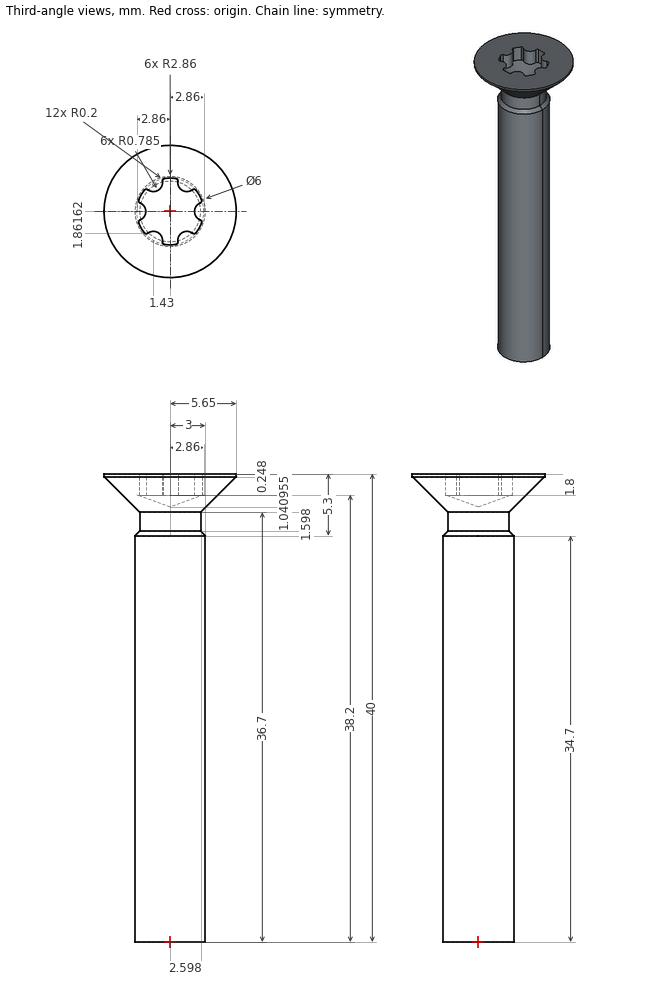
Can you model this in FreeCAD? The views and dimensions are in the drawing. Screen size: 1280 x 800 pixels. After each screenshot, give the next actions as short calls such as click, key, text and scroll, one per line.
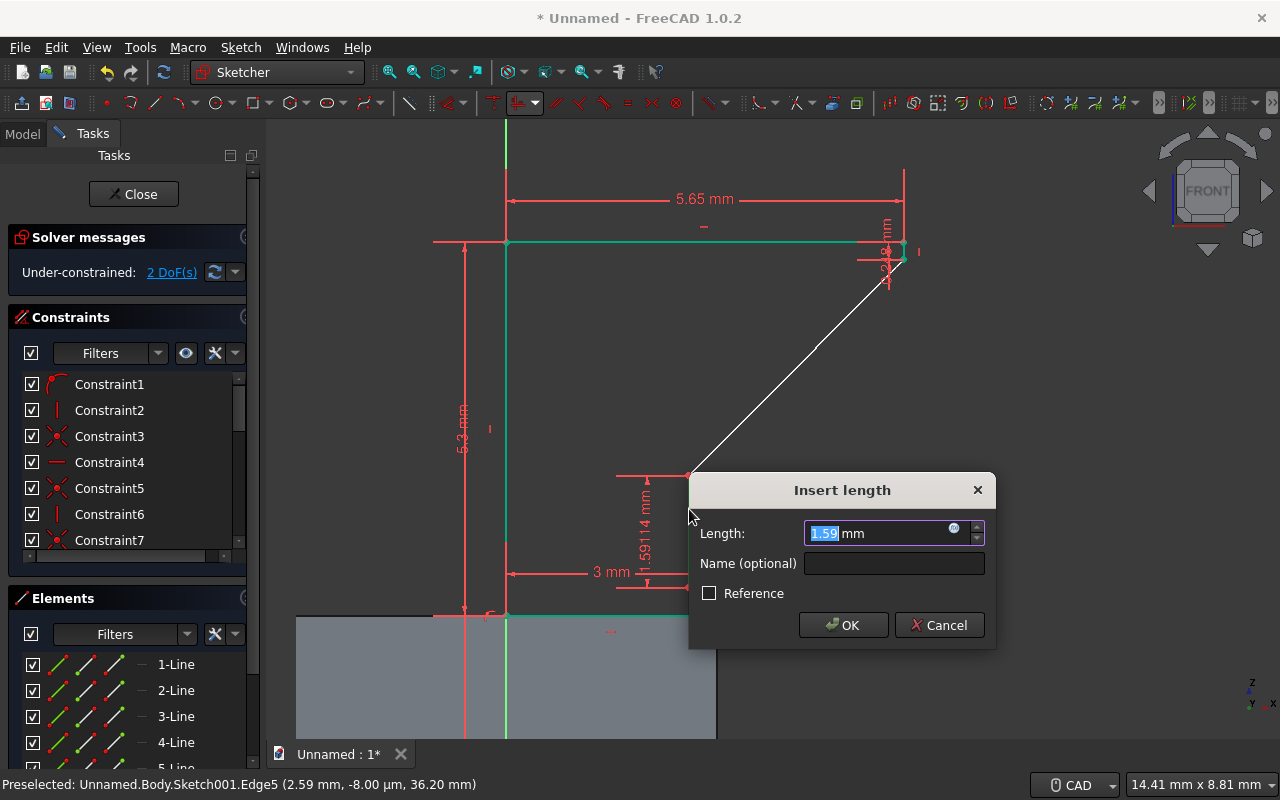
text(1.598)
key(Return)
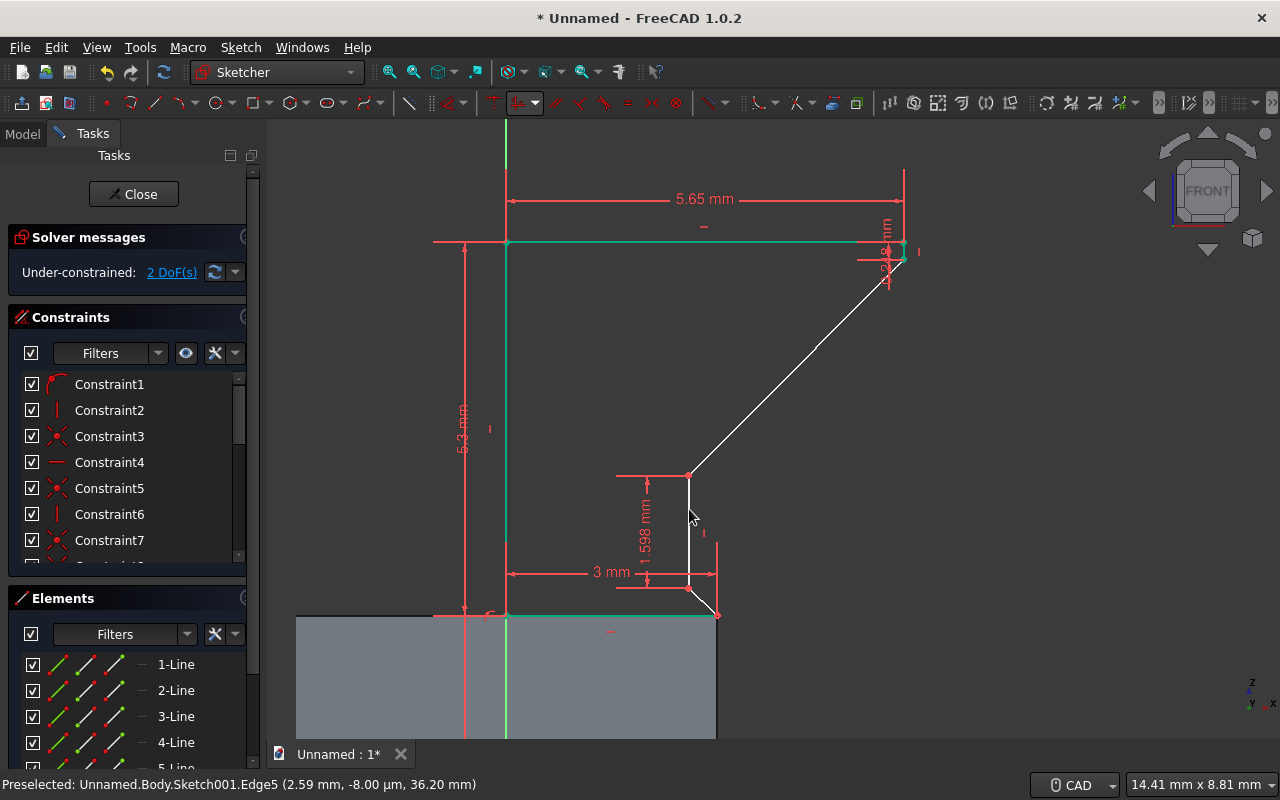
click(689, 476)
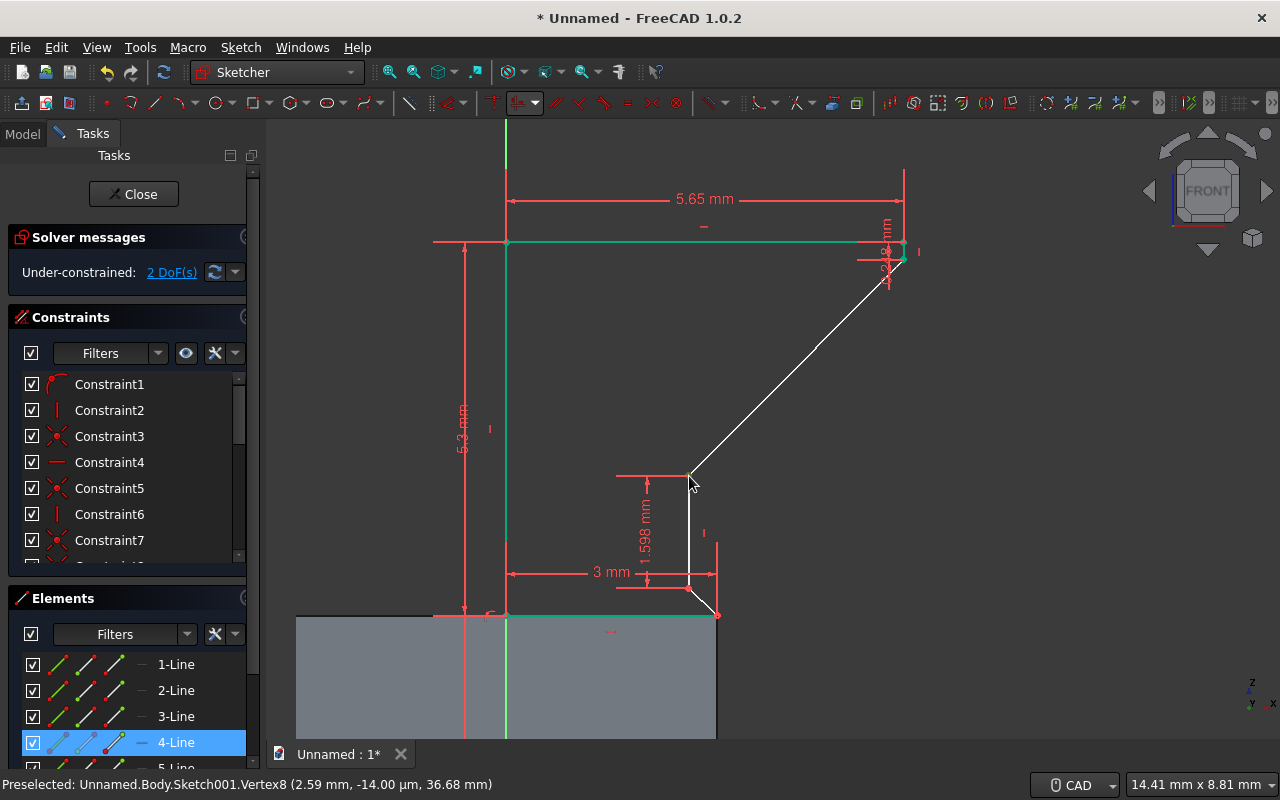
key(i)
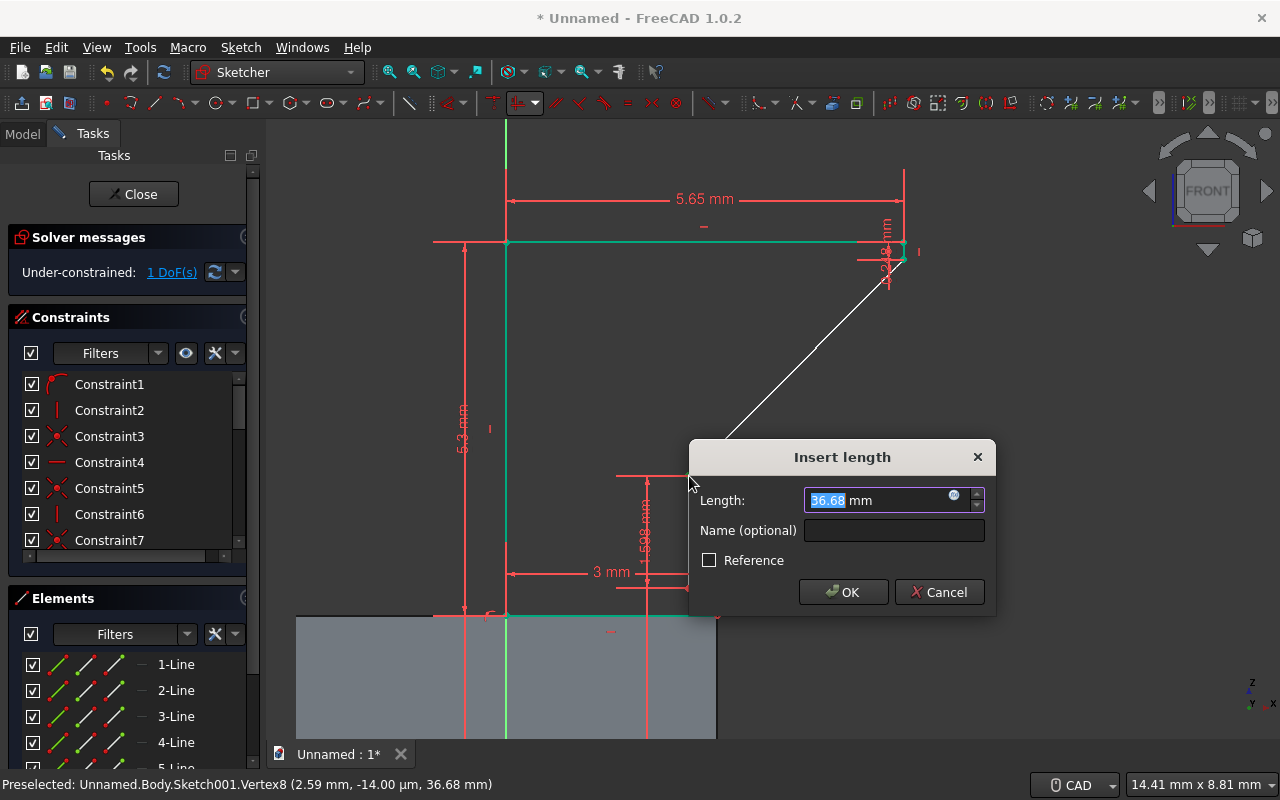
text(36.7)
key(Return)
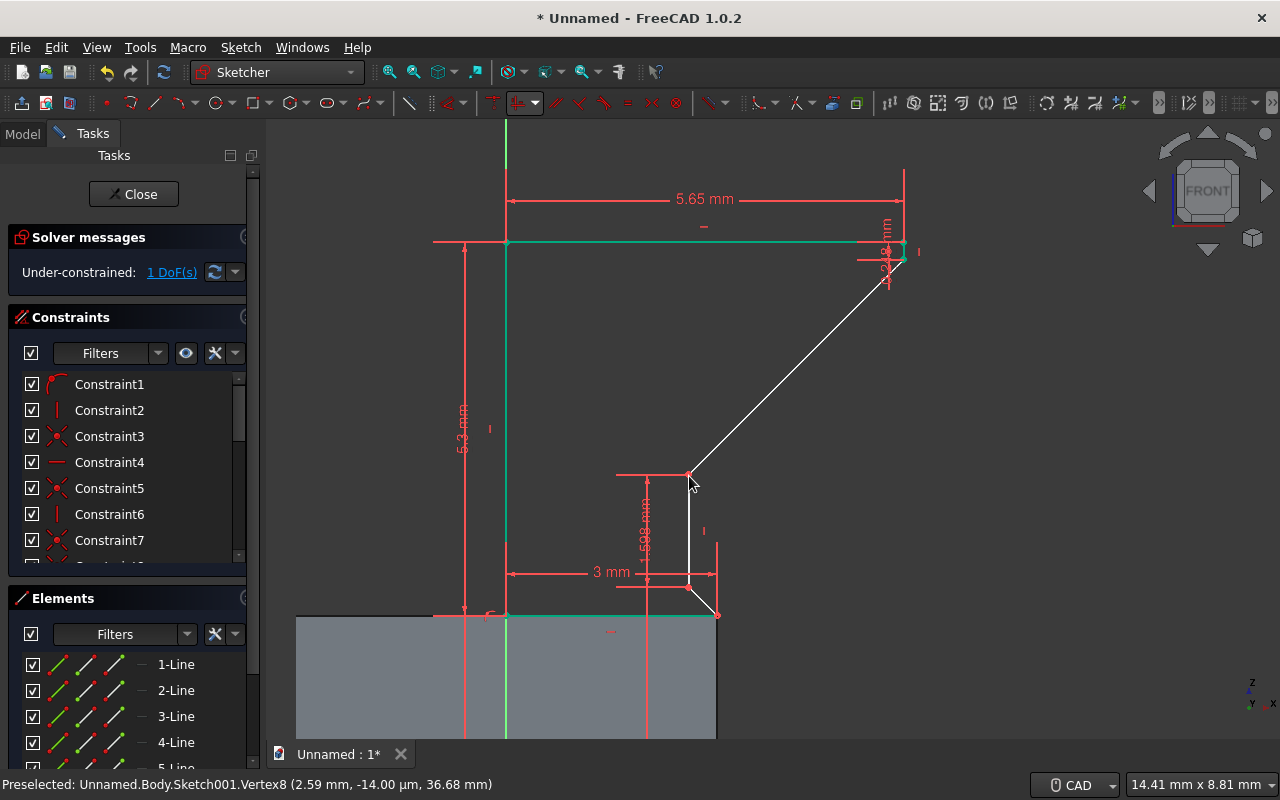
click(689, 475)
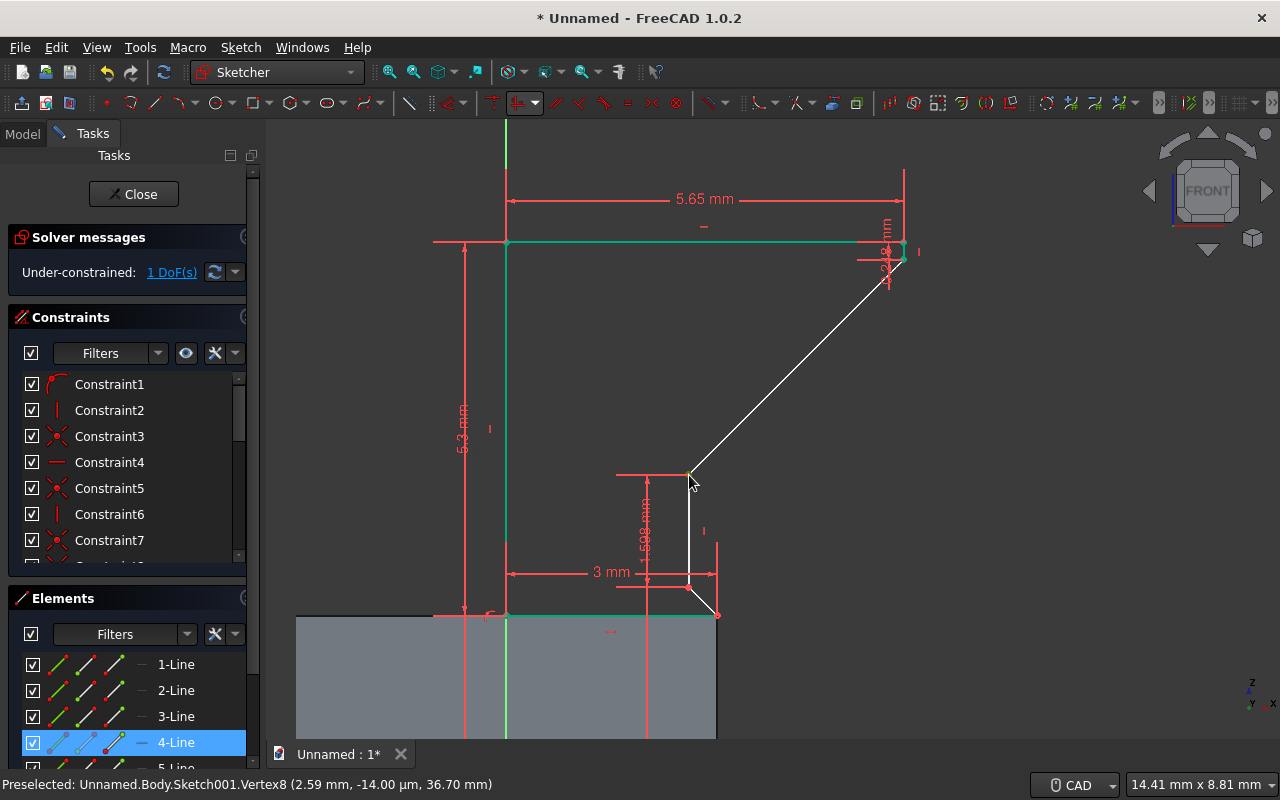
key(l)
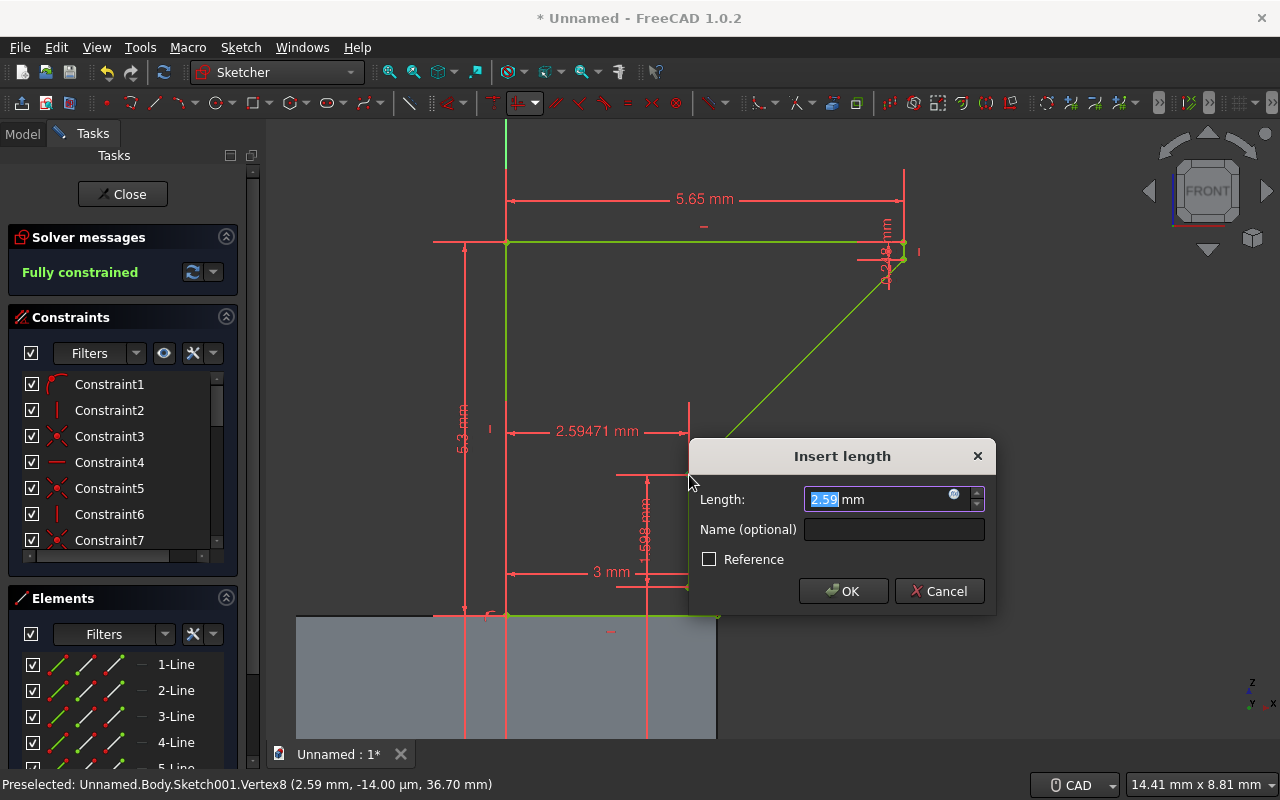
text(2.598)
key(Return)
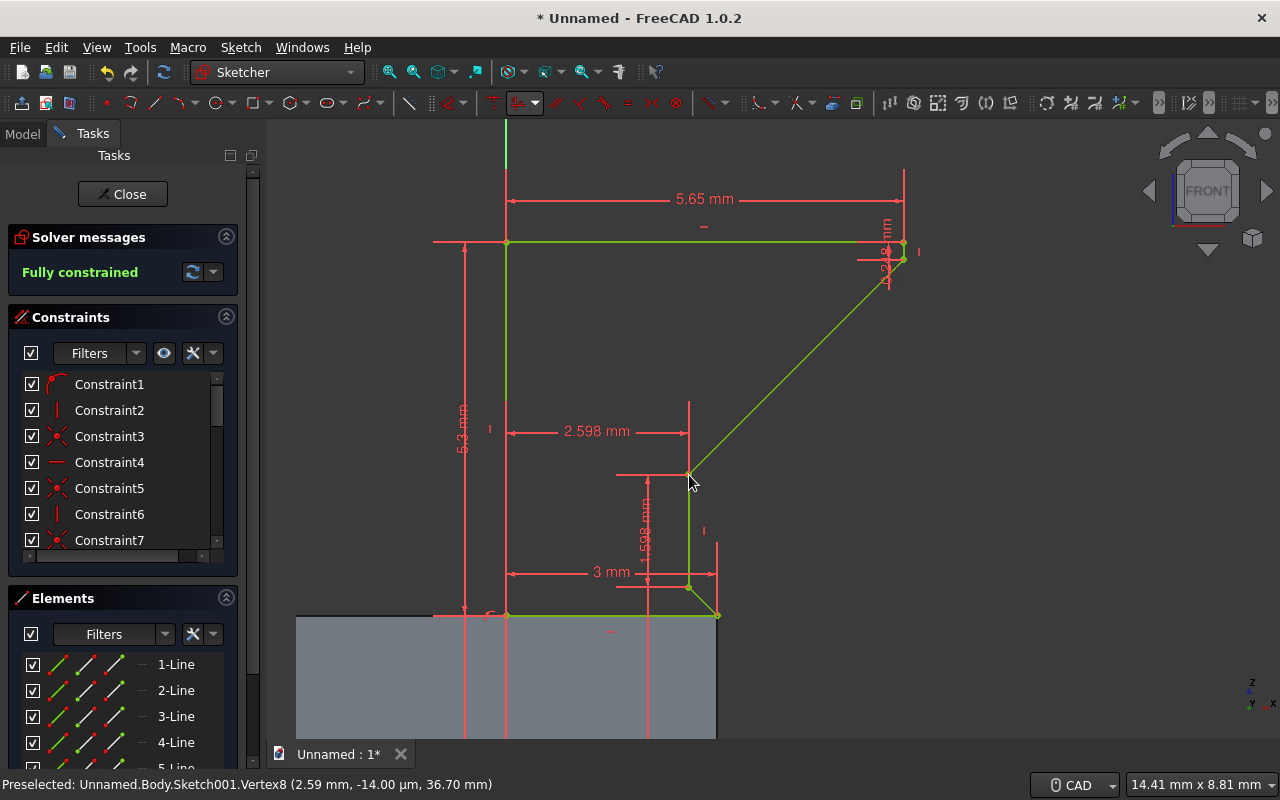
click(123, 194)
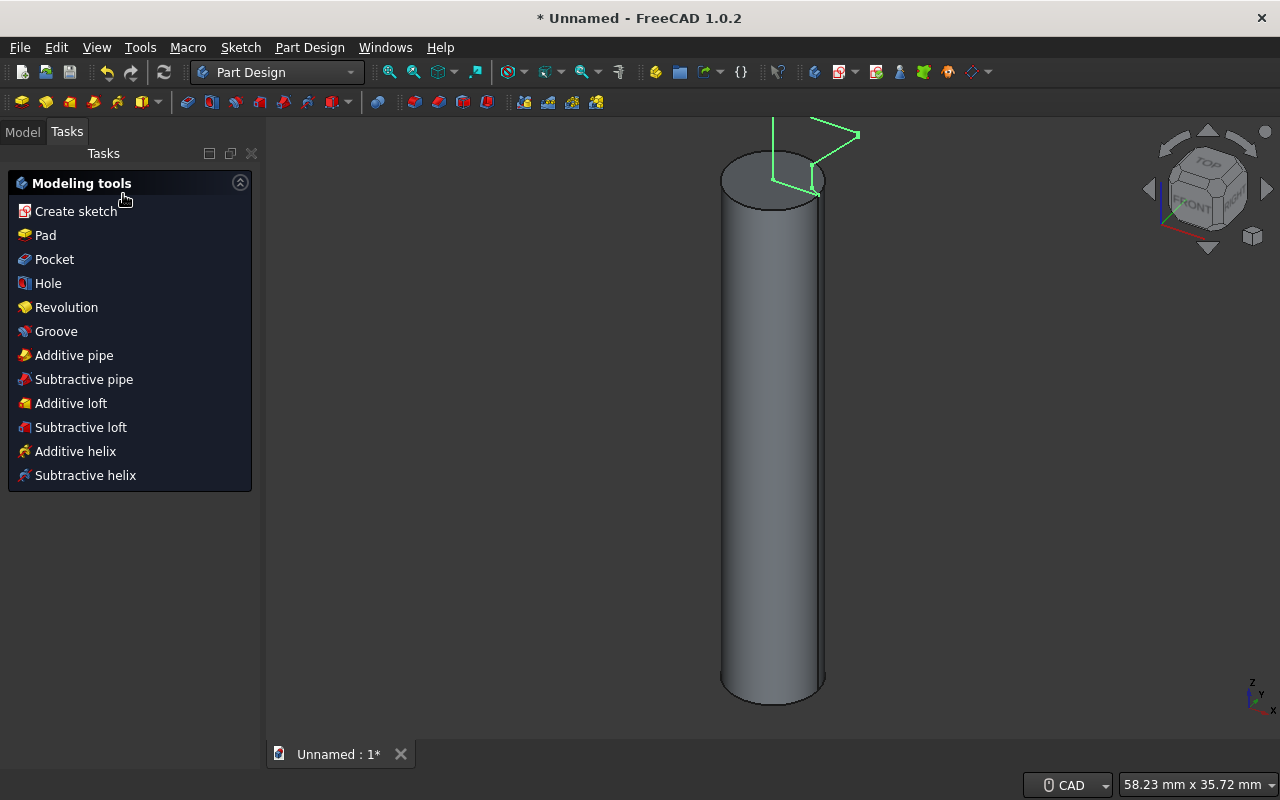
click(46, 102)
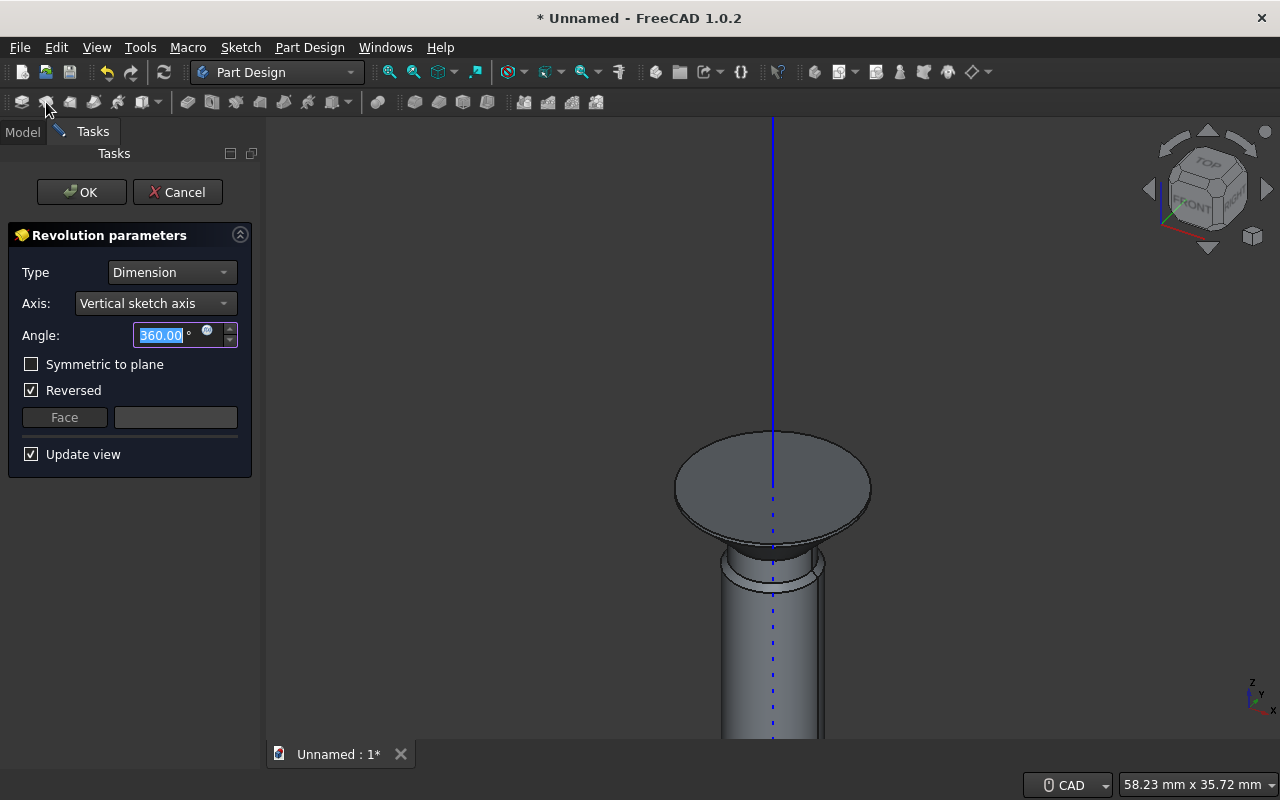
click(82, 192)